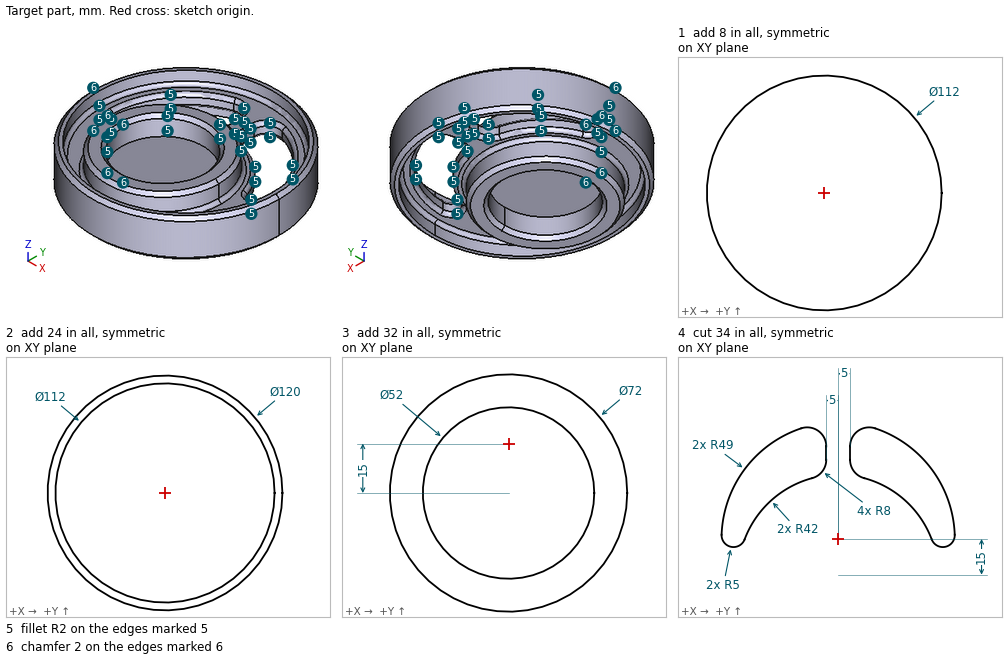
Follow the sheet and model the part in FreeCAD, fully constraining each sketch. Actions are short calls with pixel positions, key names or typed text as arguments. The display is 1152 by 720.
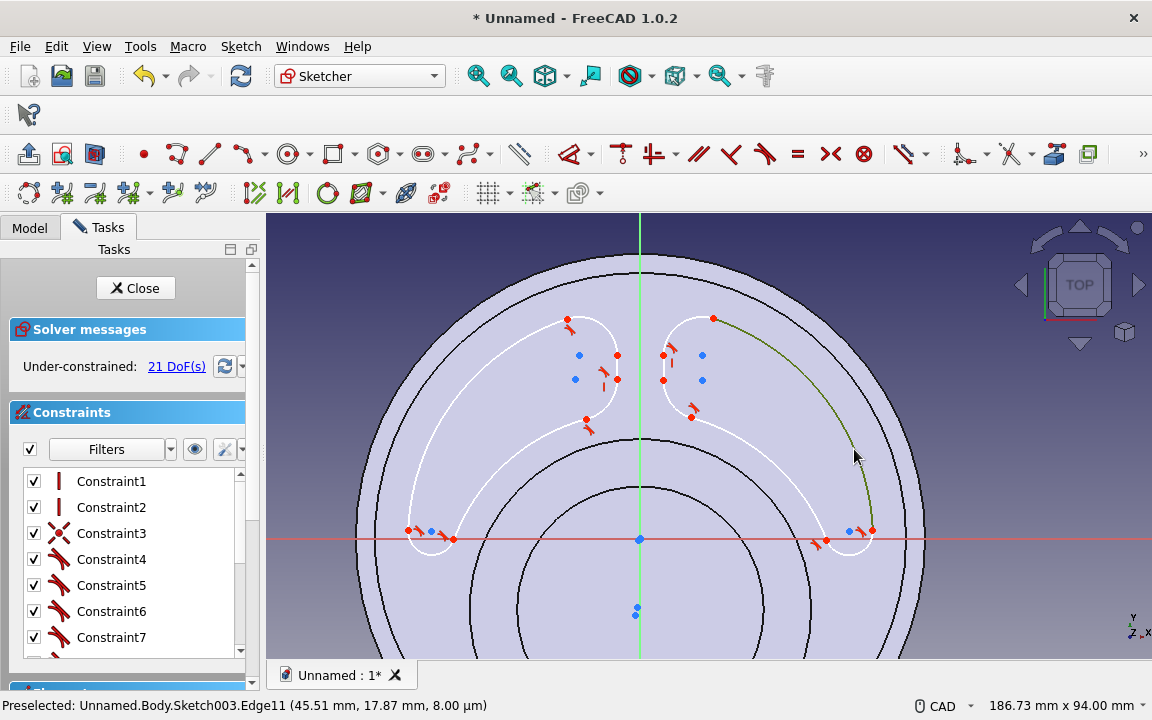
click(692, 318)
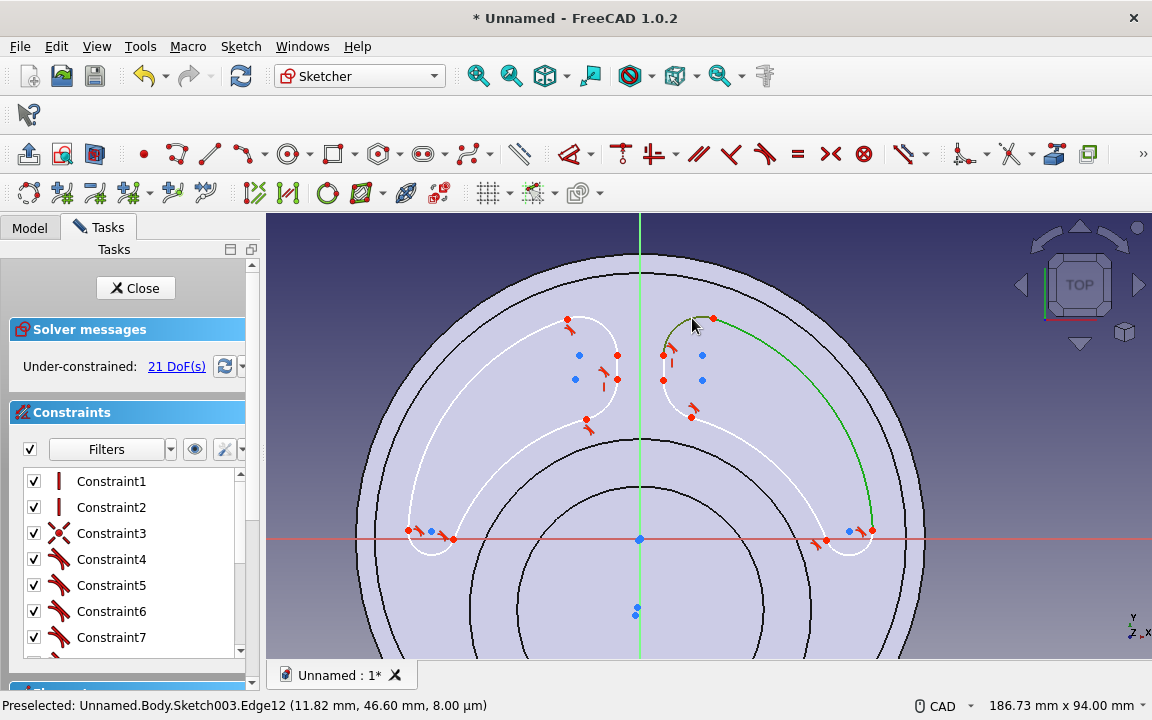
click(765, 154)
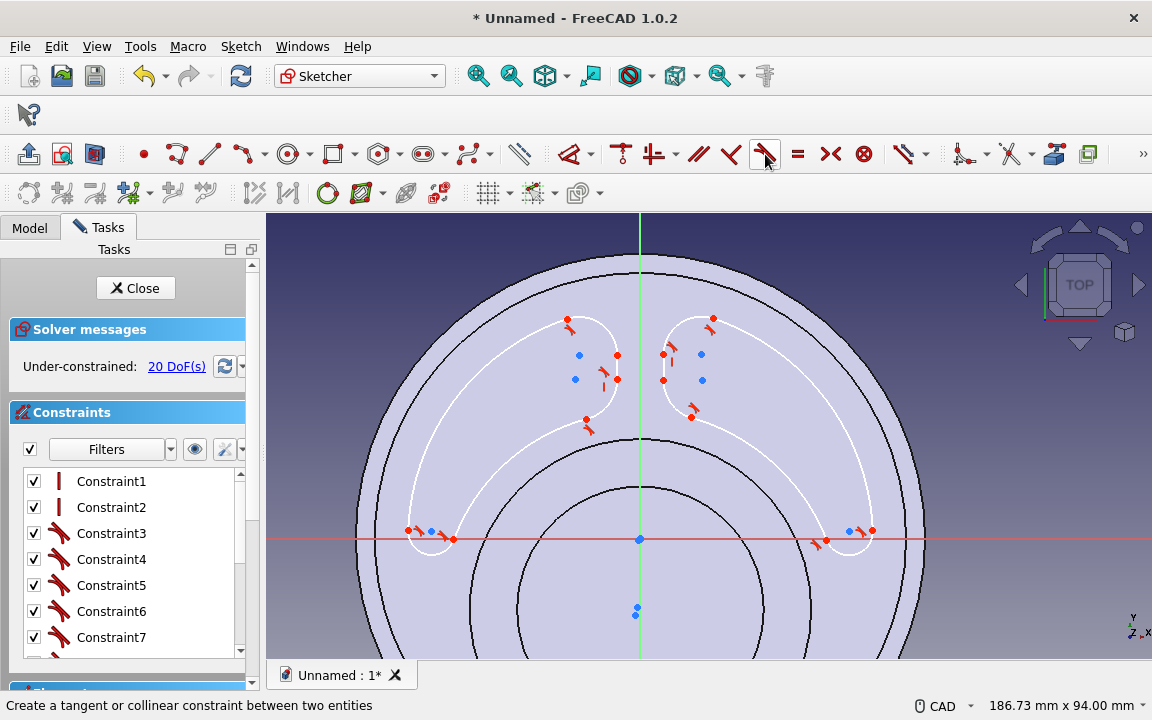
click(535, 441)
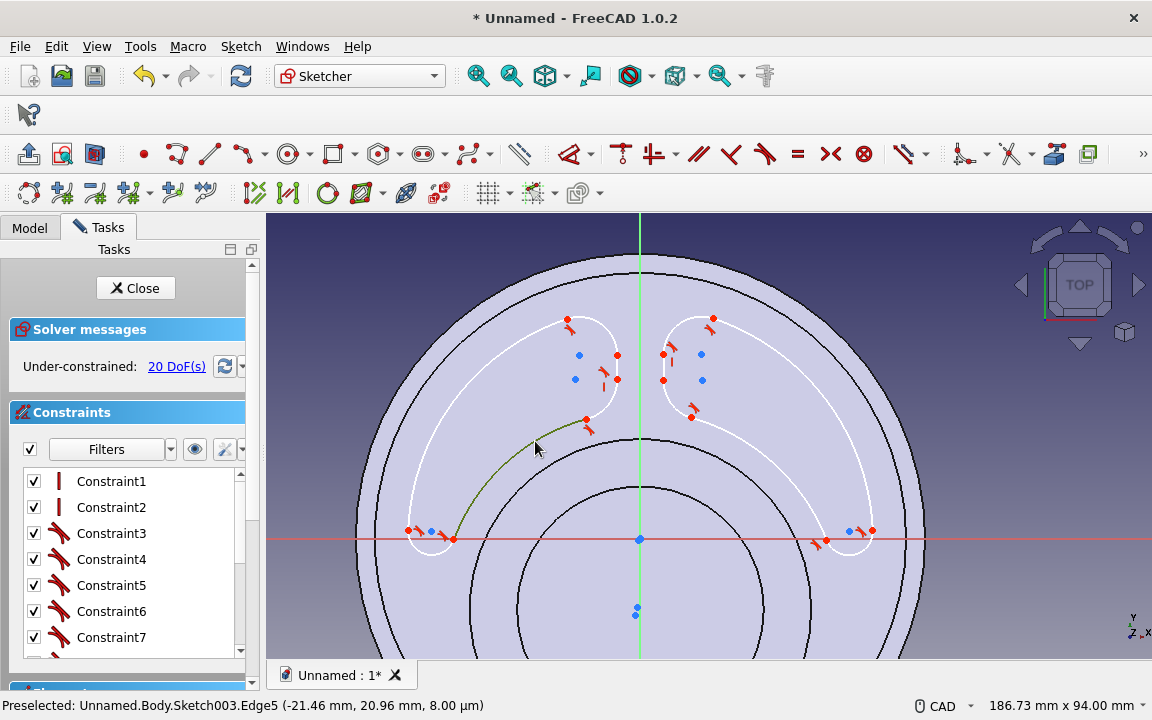
click(799, 491)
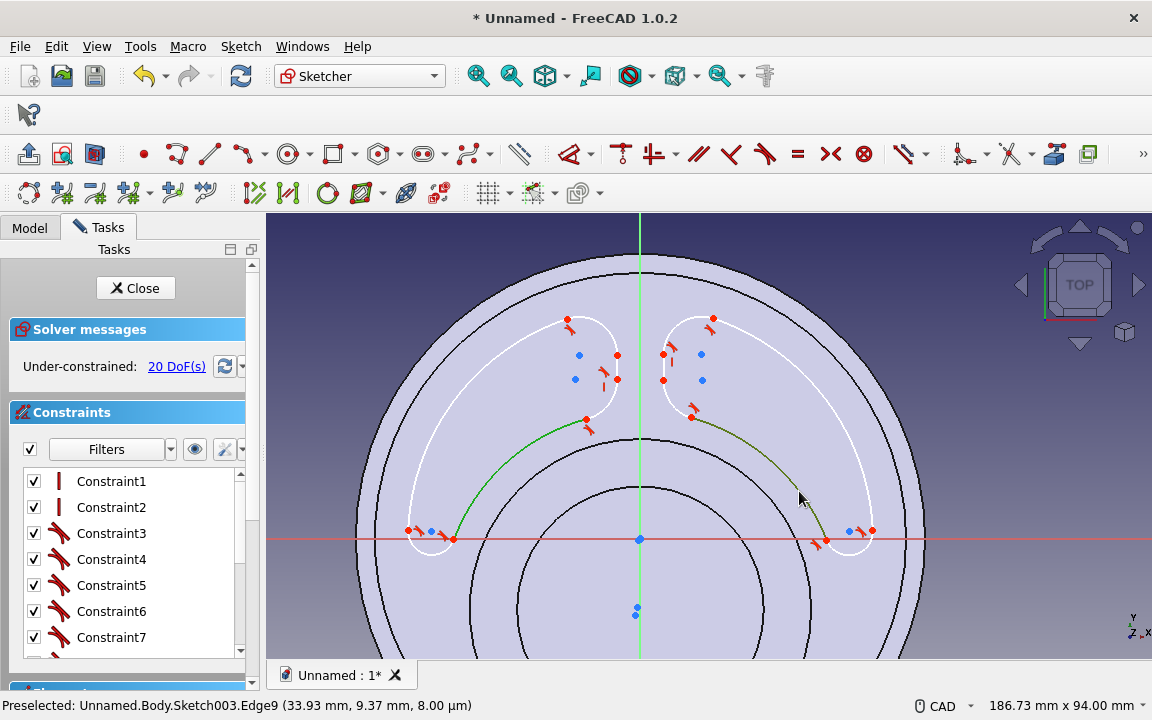
key(c)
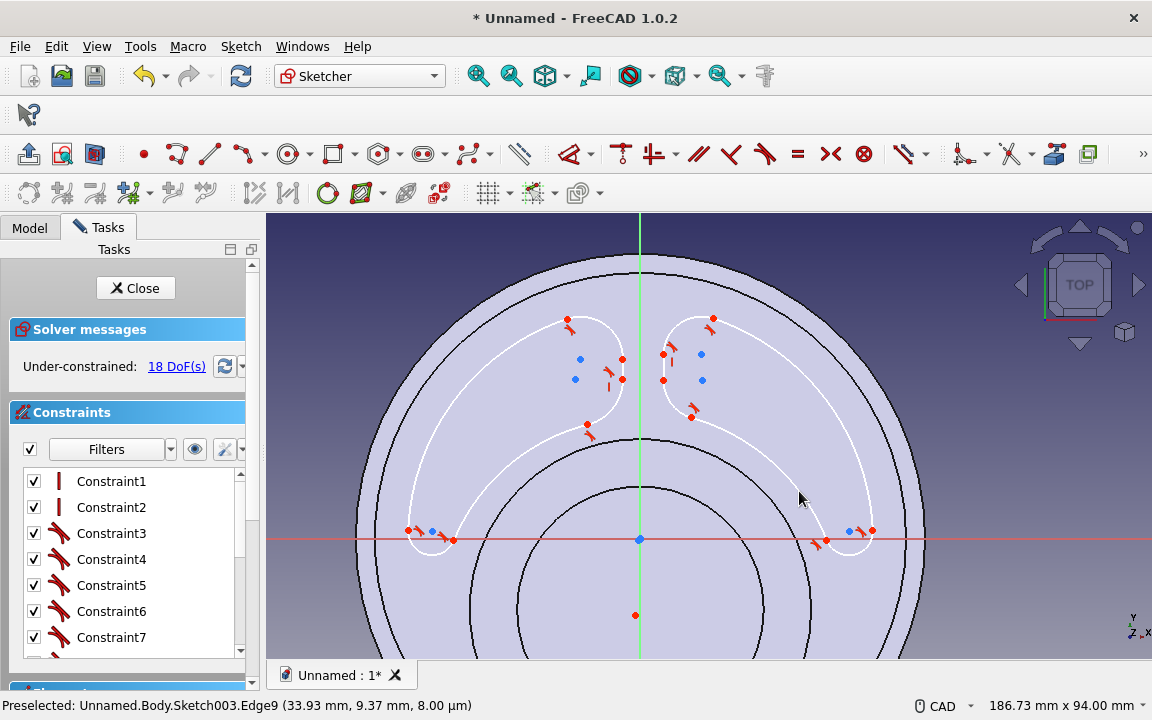
click(494, 359)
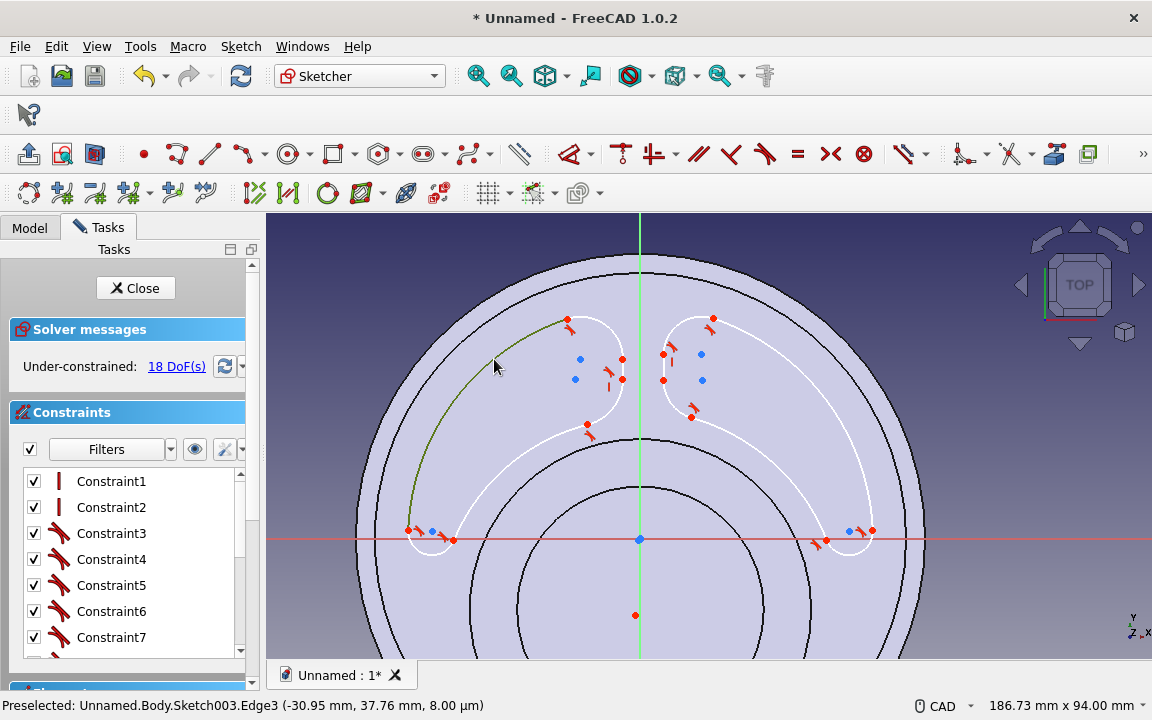
click(854, 449)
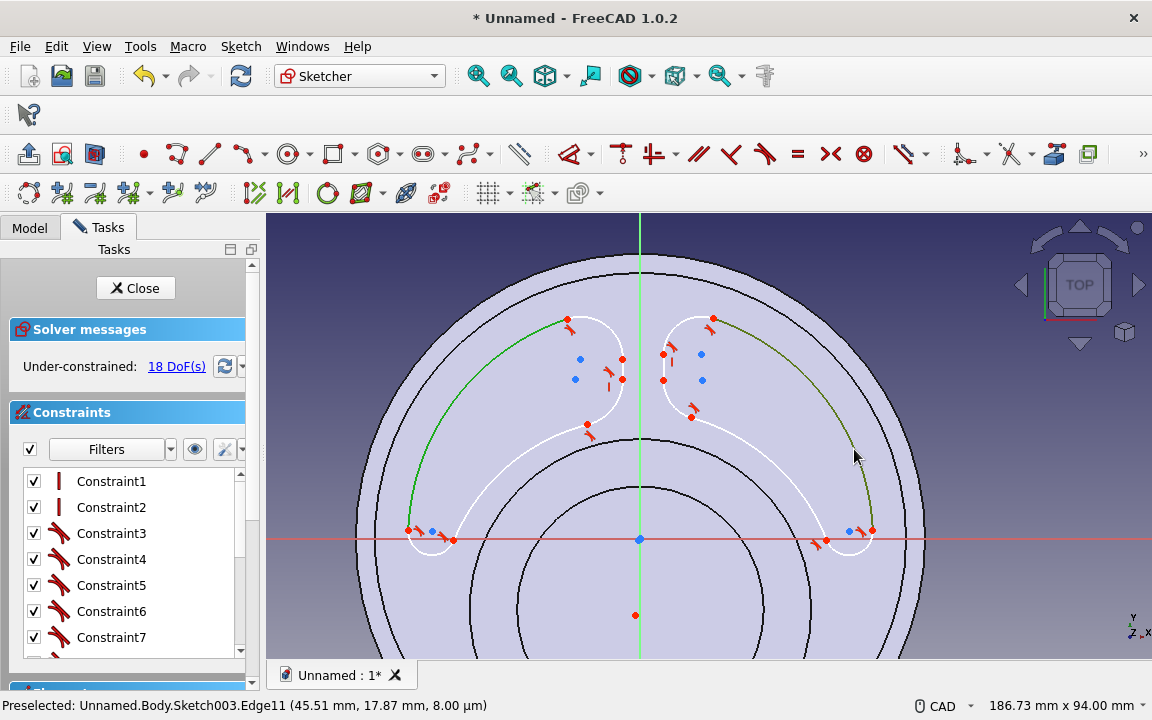
click(621, 154)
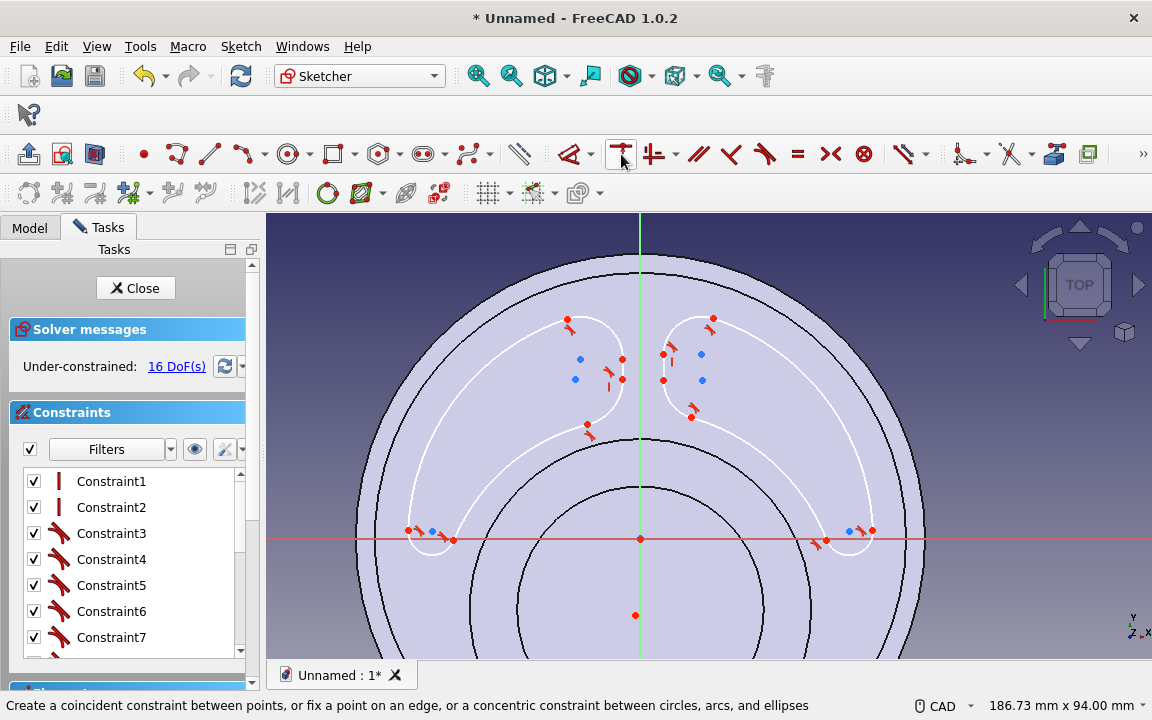
scroll(640, 539, up, 3)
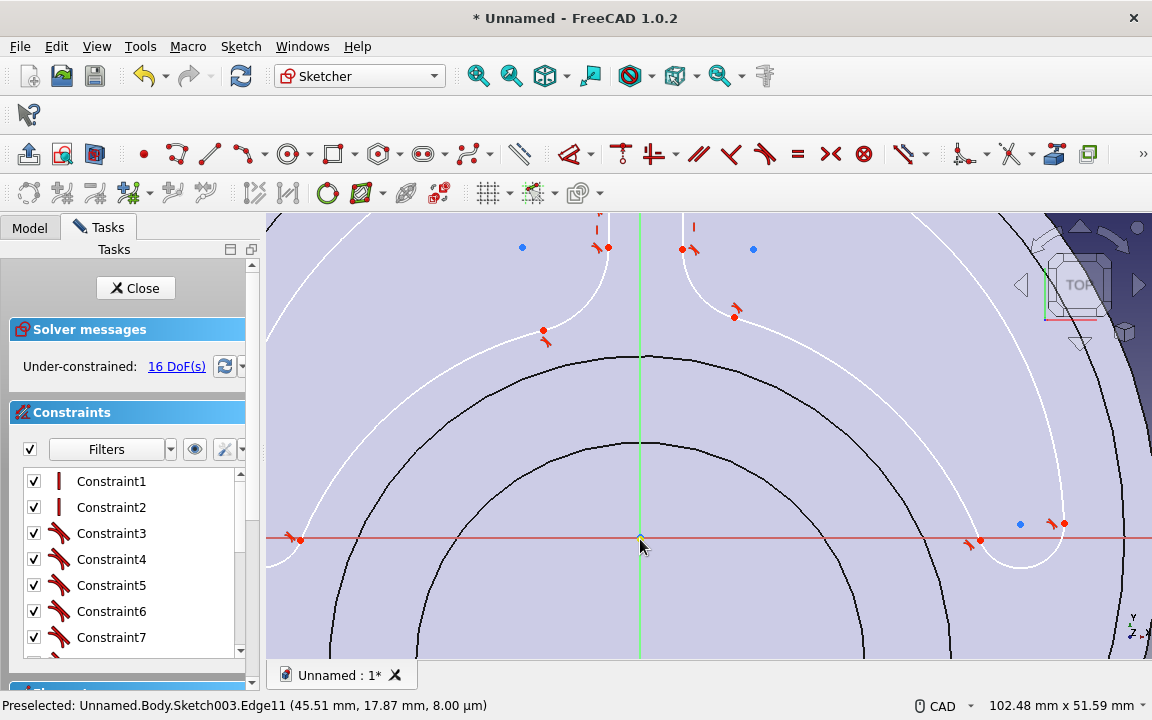
drag(630, 528, 650, 549)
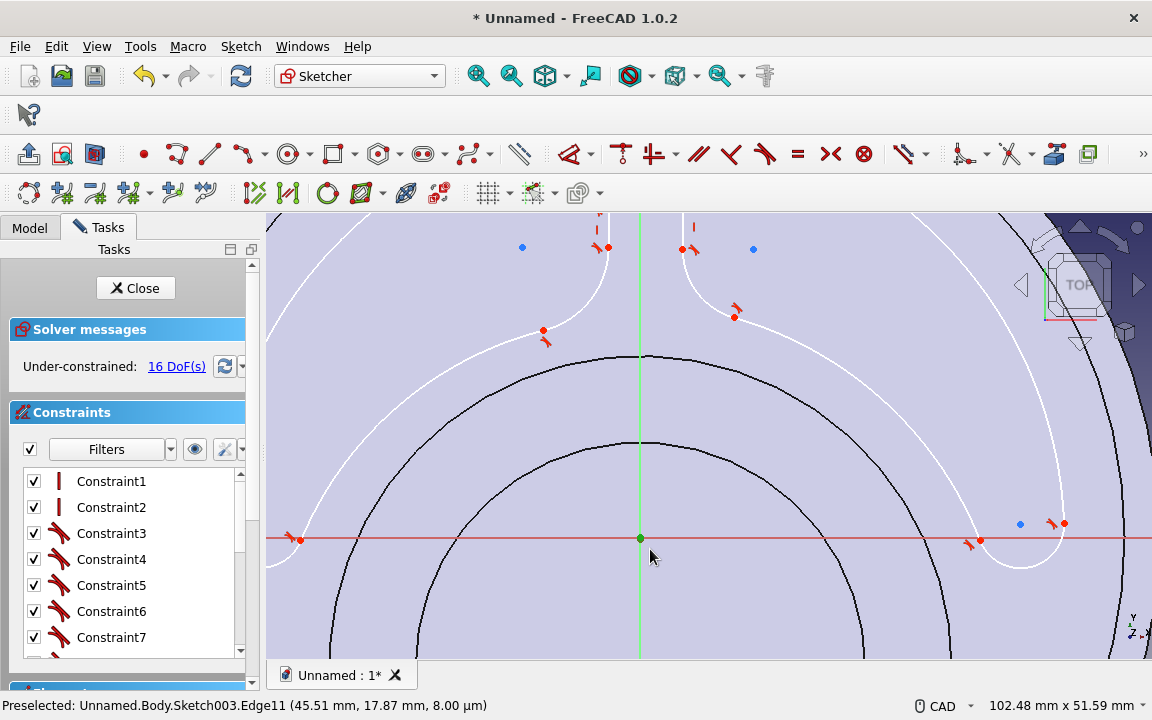
click(621, 154)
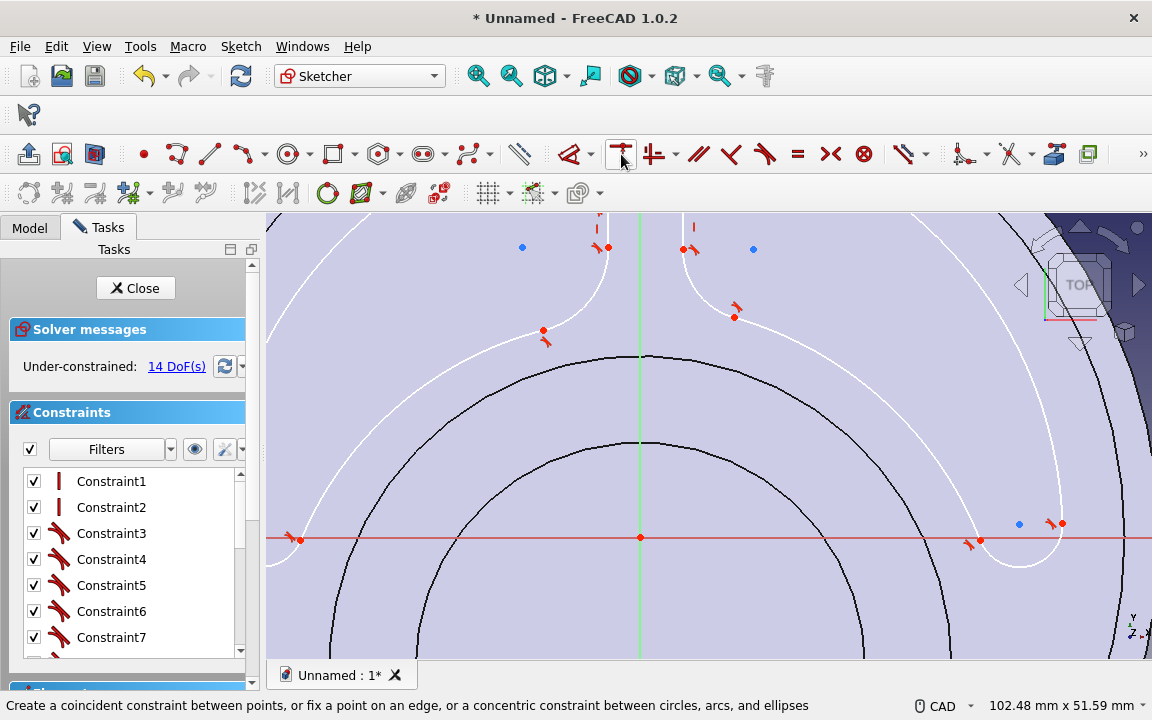
scroll(641, 539, down, 3)